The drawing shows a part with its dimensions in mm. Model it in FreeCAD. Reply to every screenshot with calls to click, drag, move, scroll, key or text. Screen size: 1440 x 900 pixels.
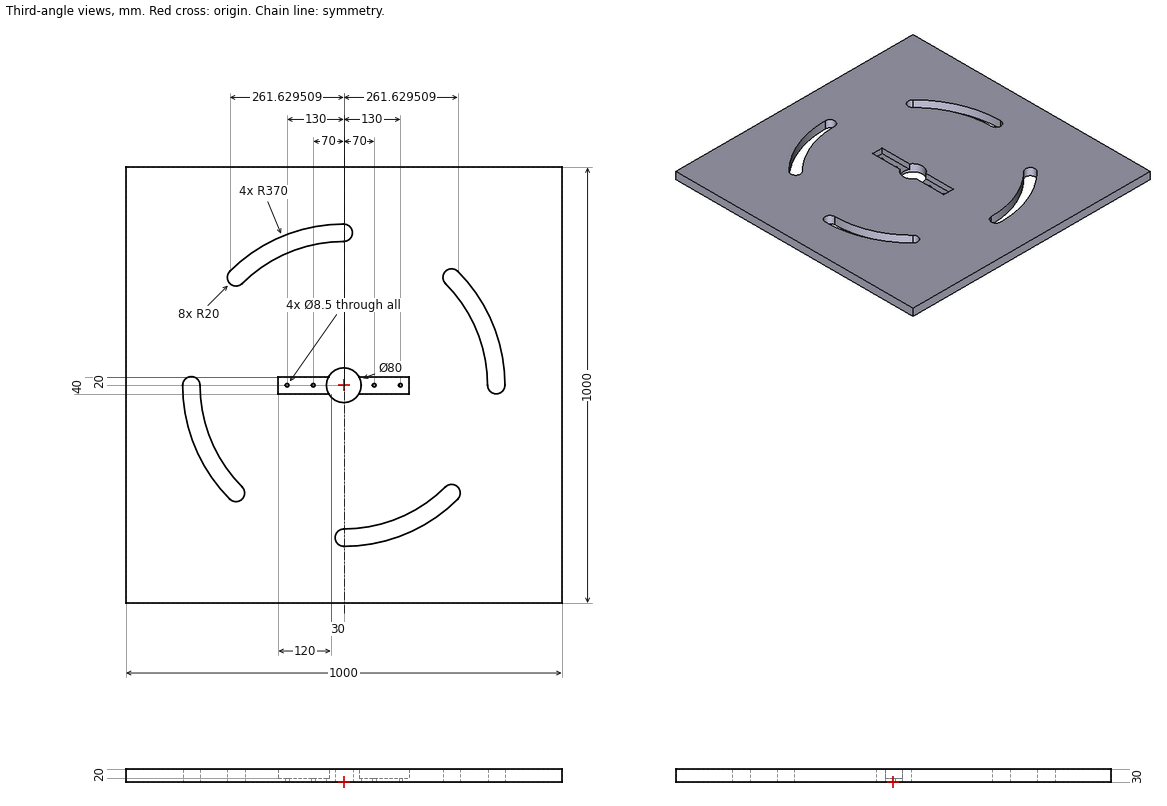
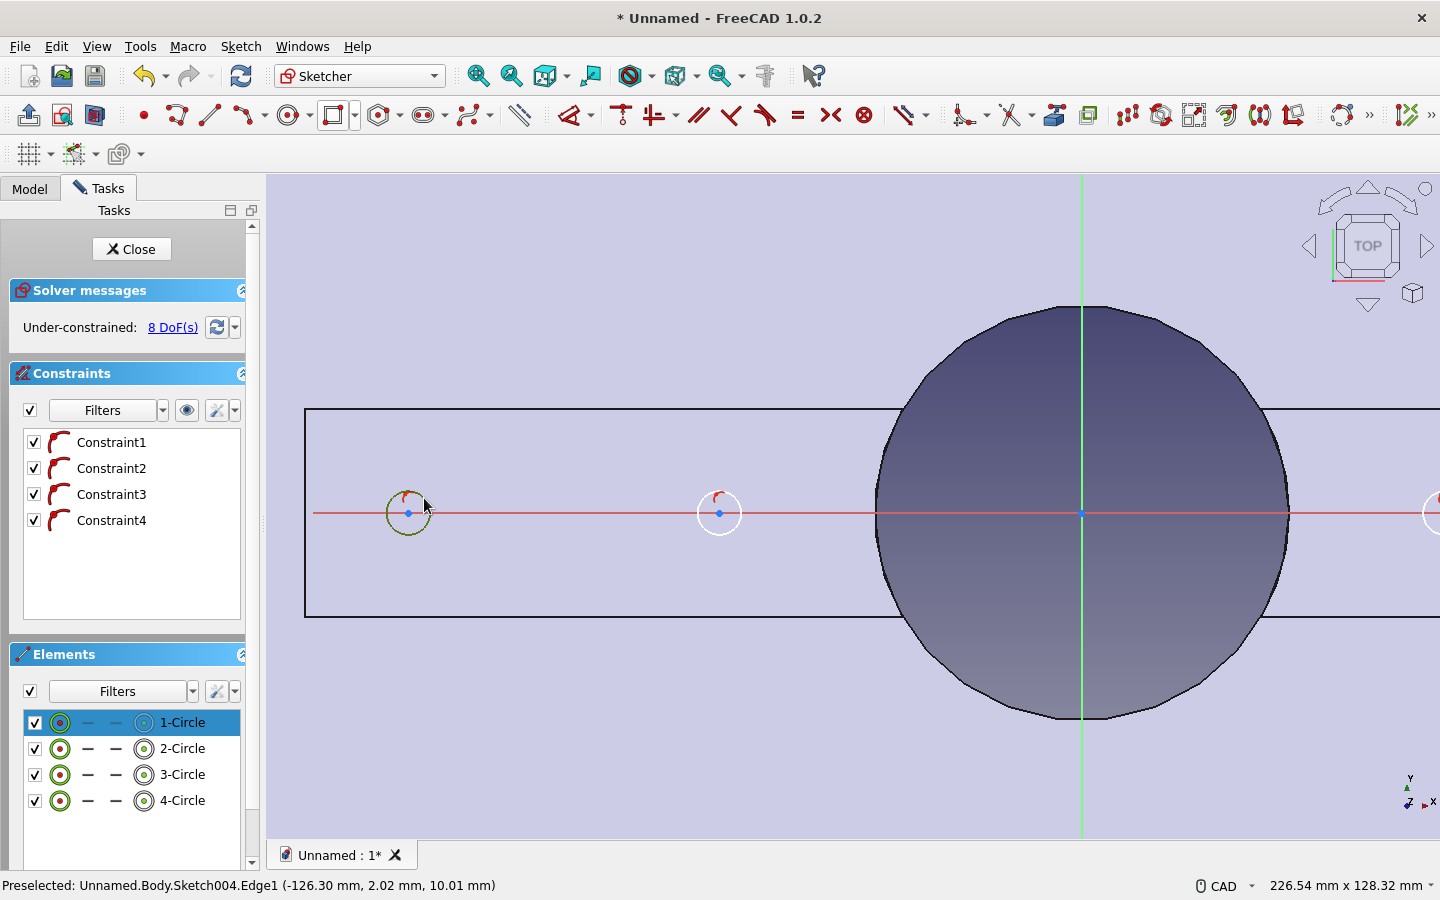
click(735, 498)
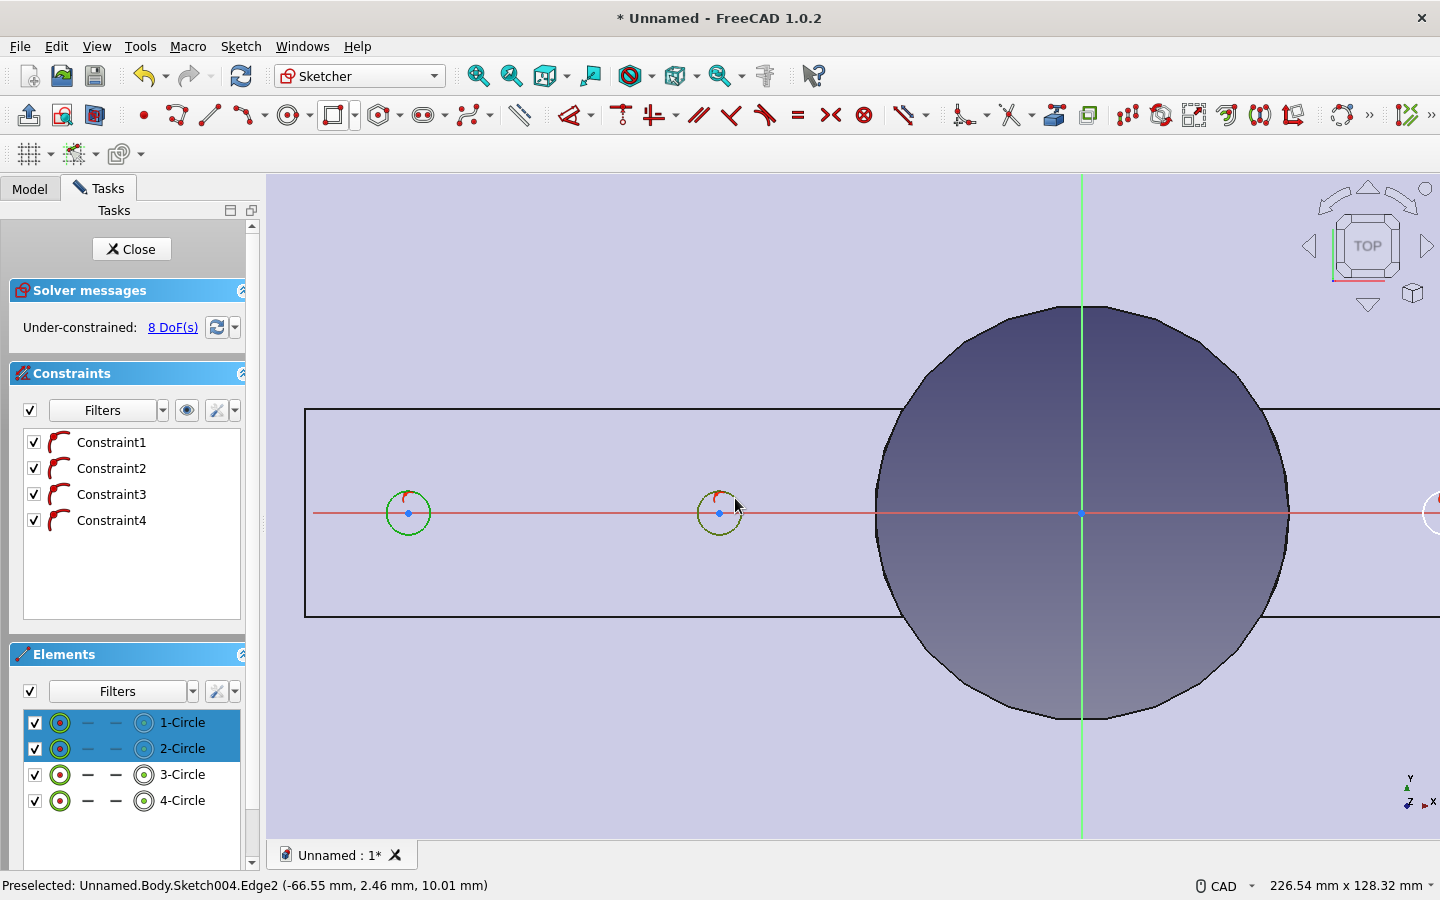
scroll(423, 498, down, 3)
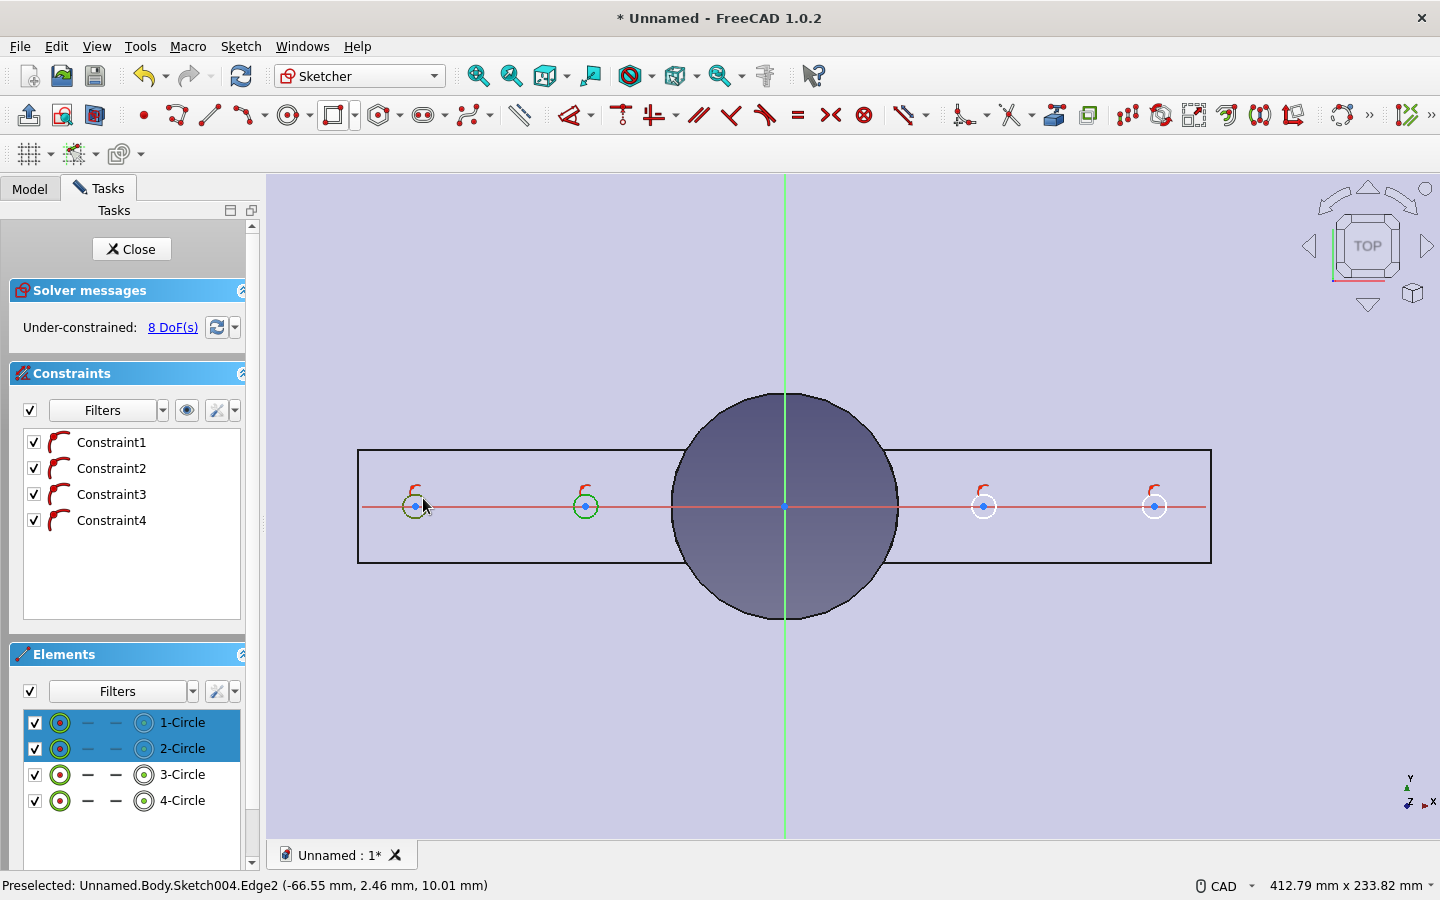
scroll(992, 498, up, 3)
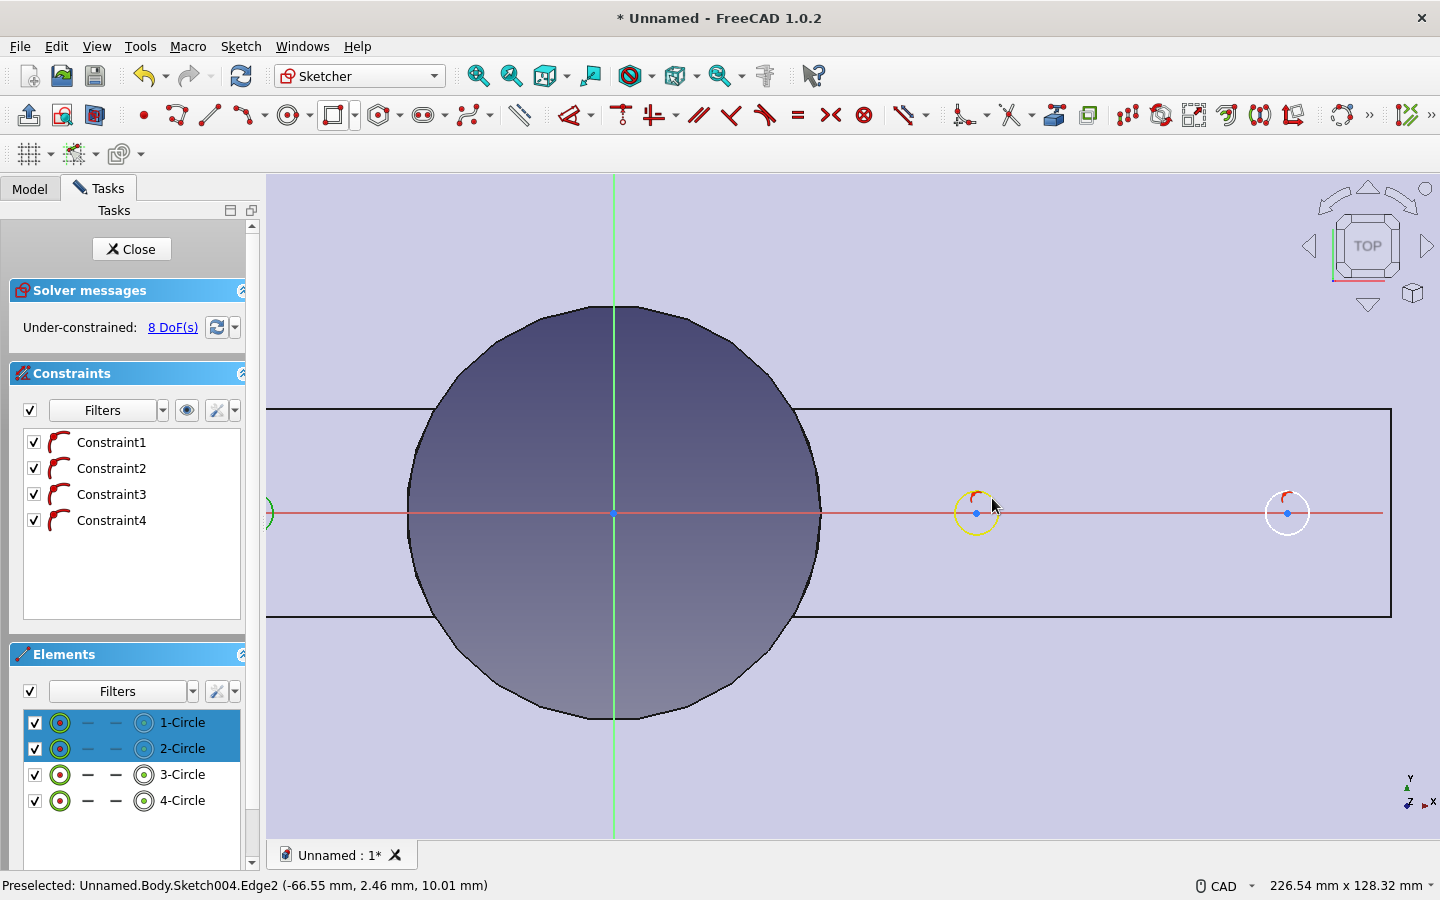
click(992, 498)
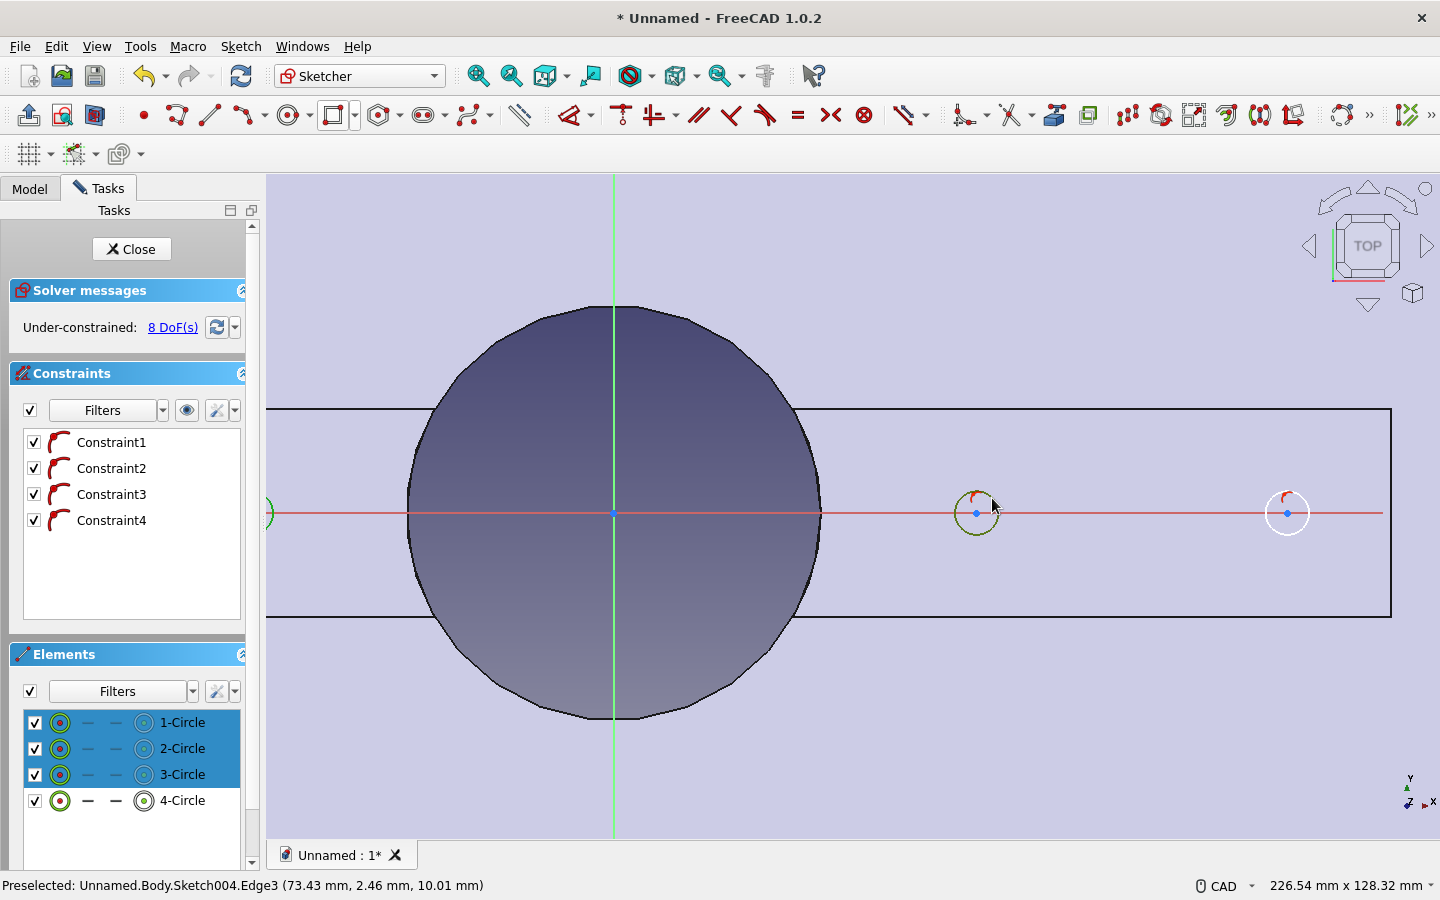
click(1272, 498)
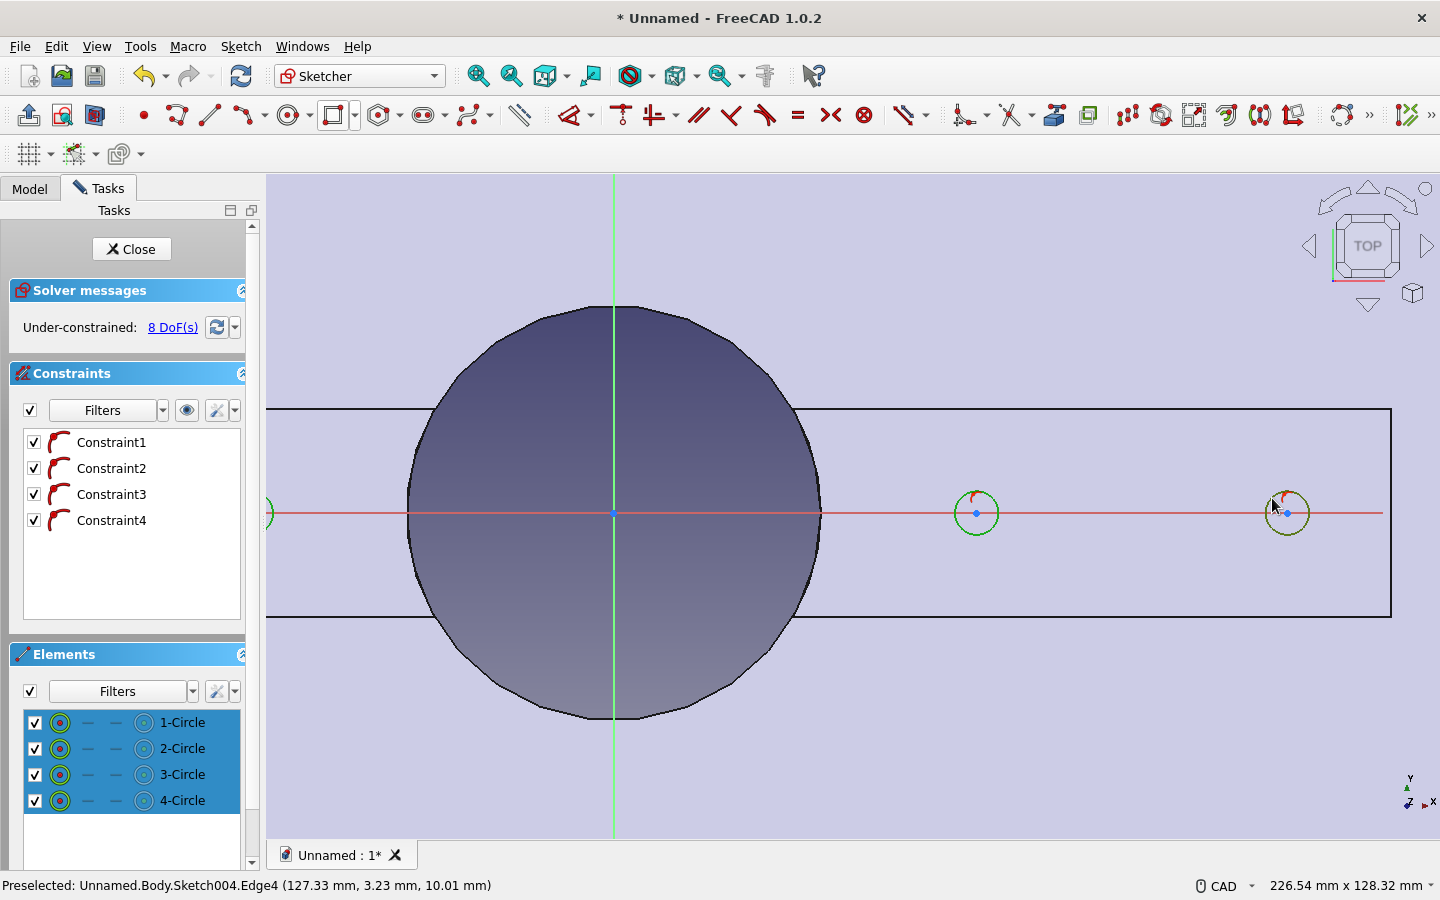
click(798, 116)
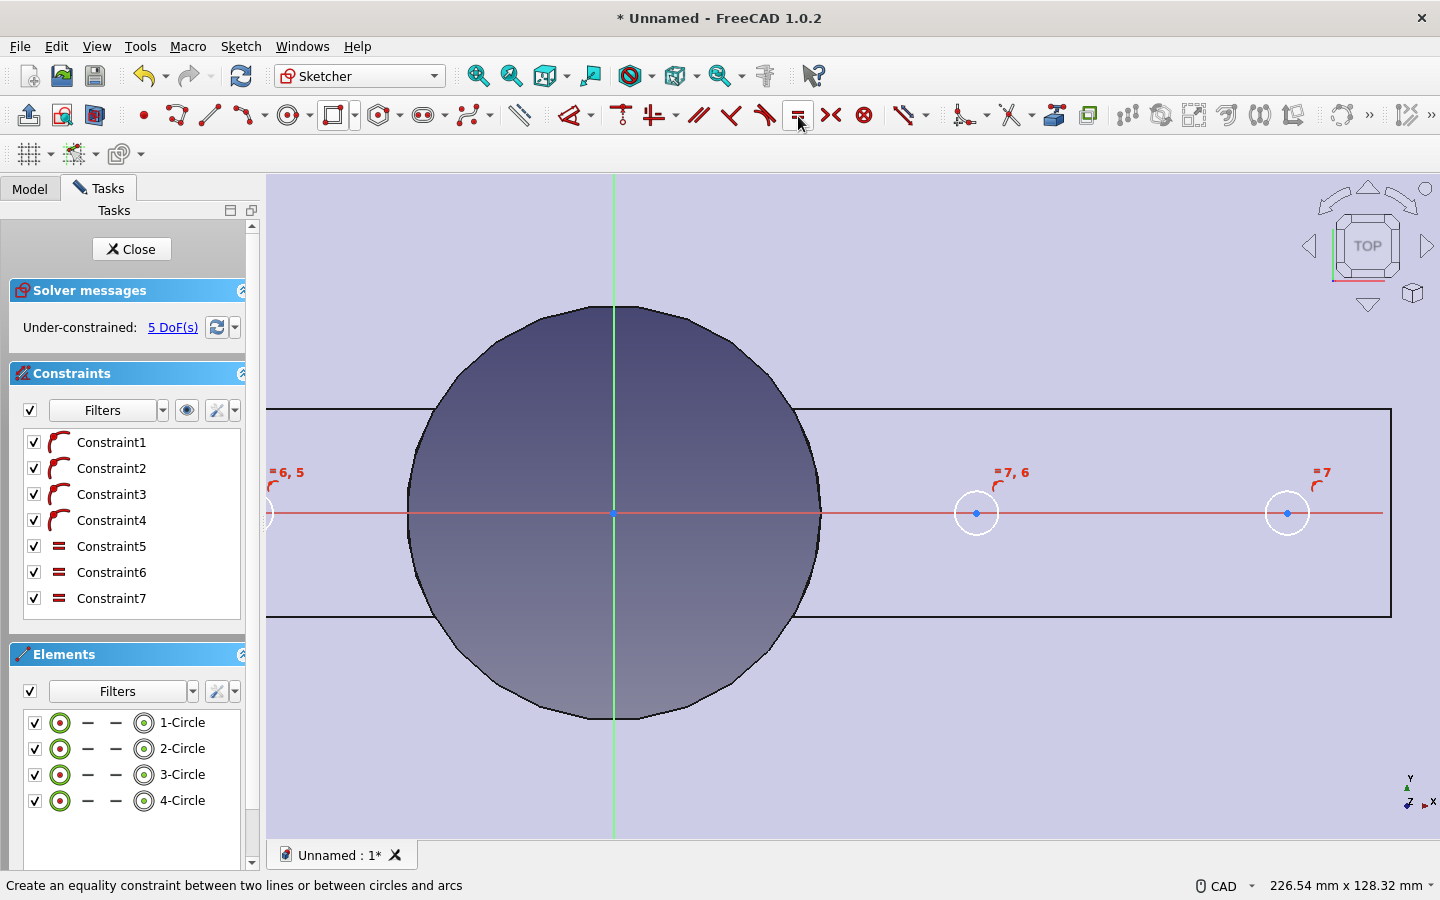
click(568, 116)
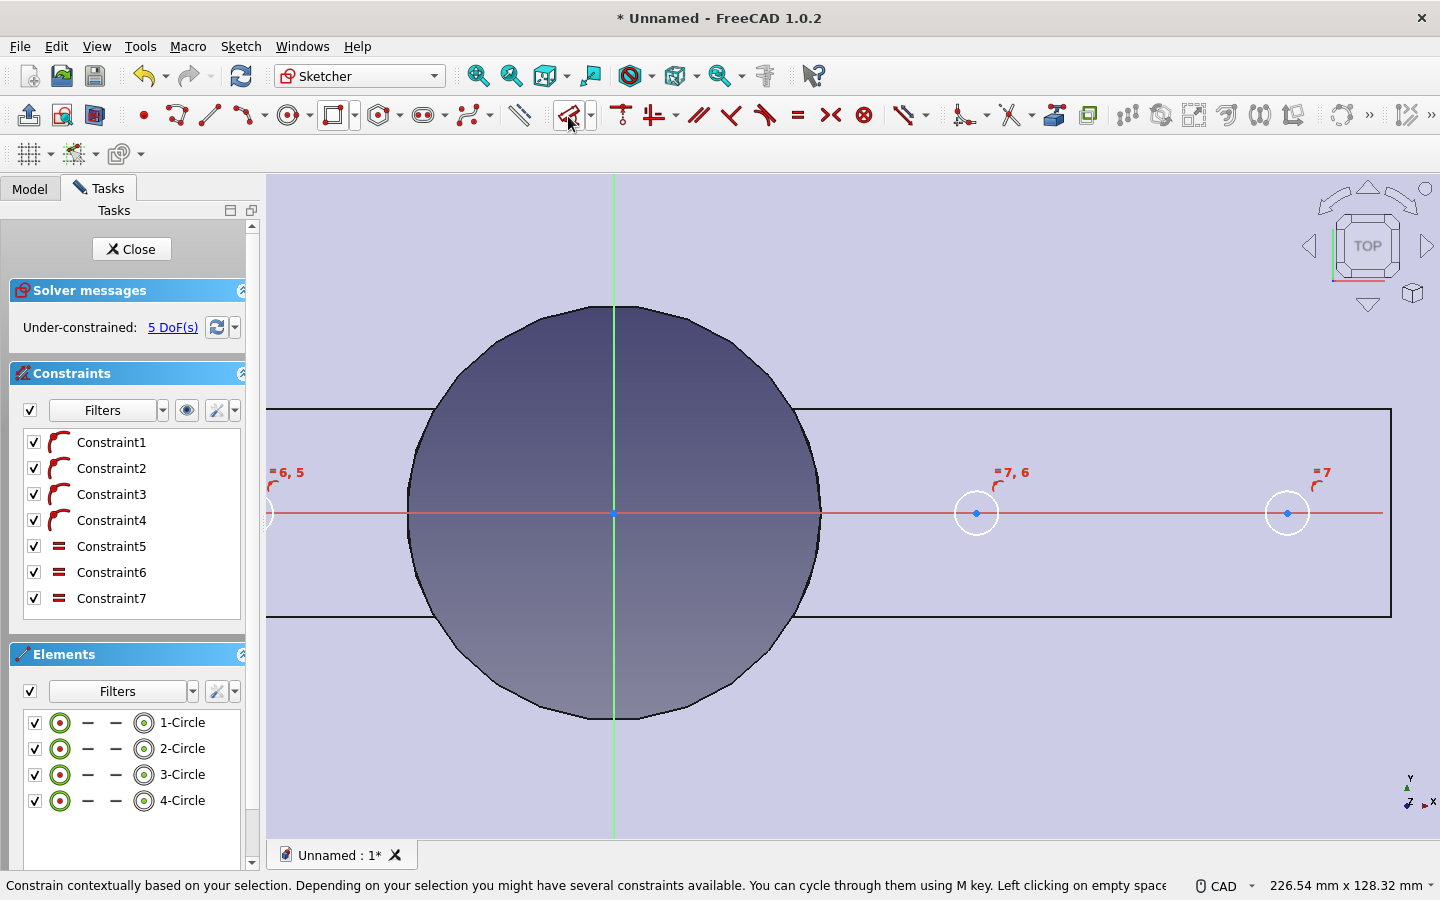
scroll(992, 498, down, 3)